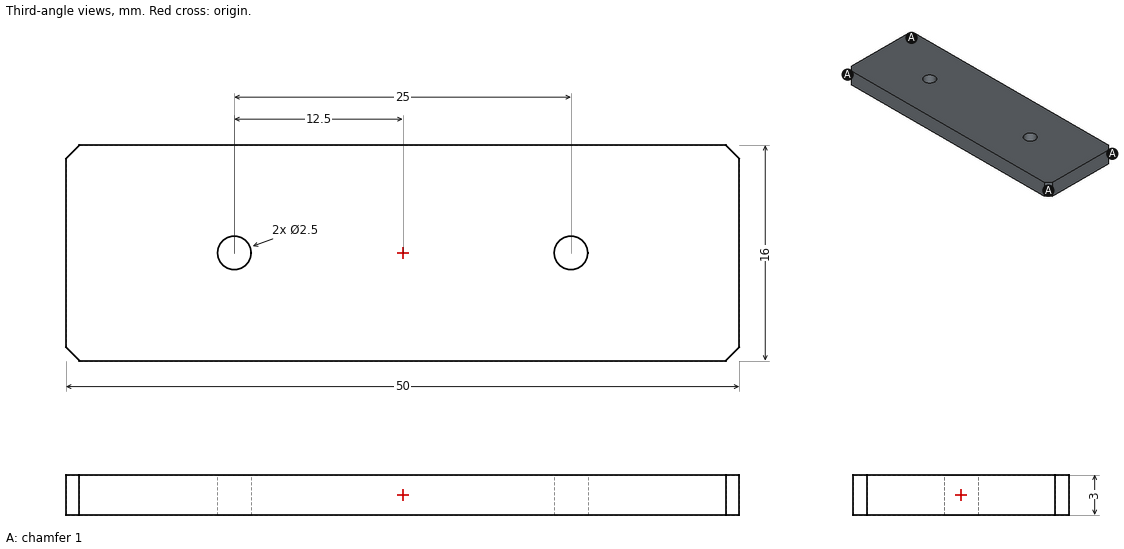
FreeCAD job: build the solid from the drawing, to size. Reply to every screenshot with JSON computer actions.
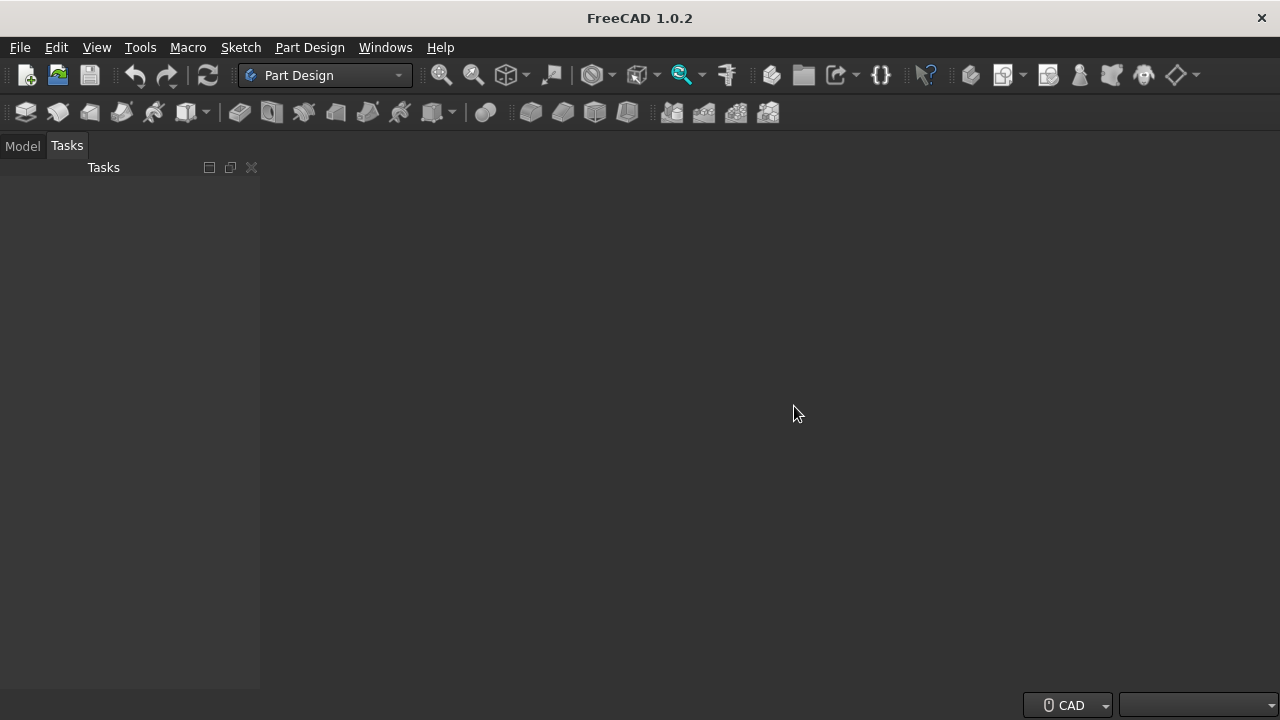
{"action": "left_click", "coordinate": [26, 76]}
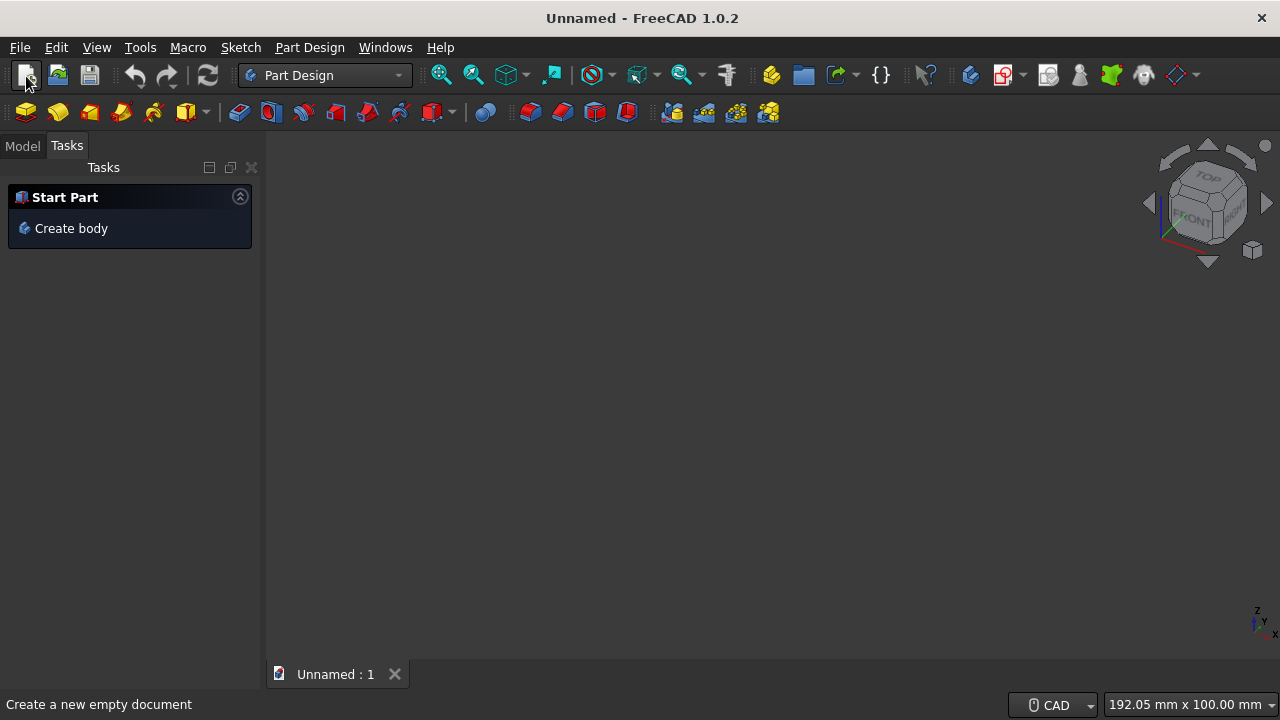
{"action": "left_click", "coordinate": [1004, 76]}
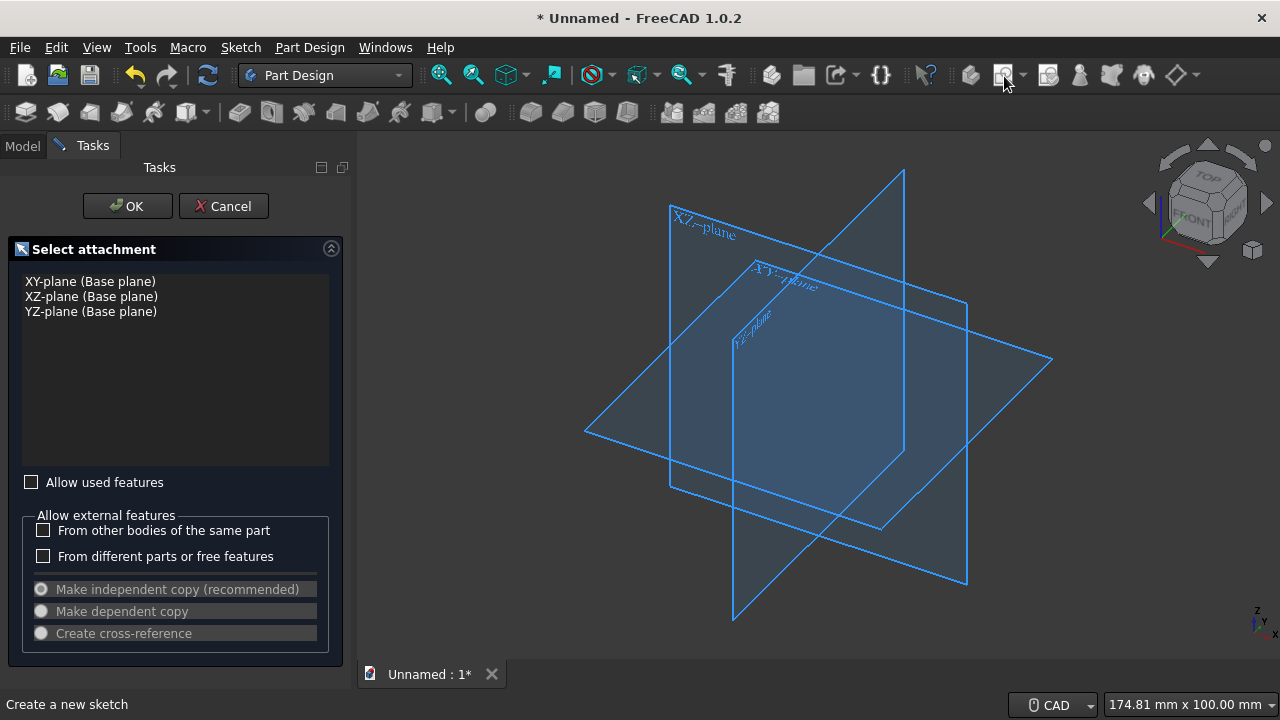
{"action": "left_click", "coordinate": [82, 282]}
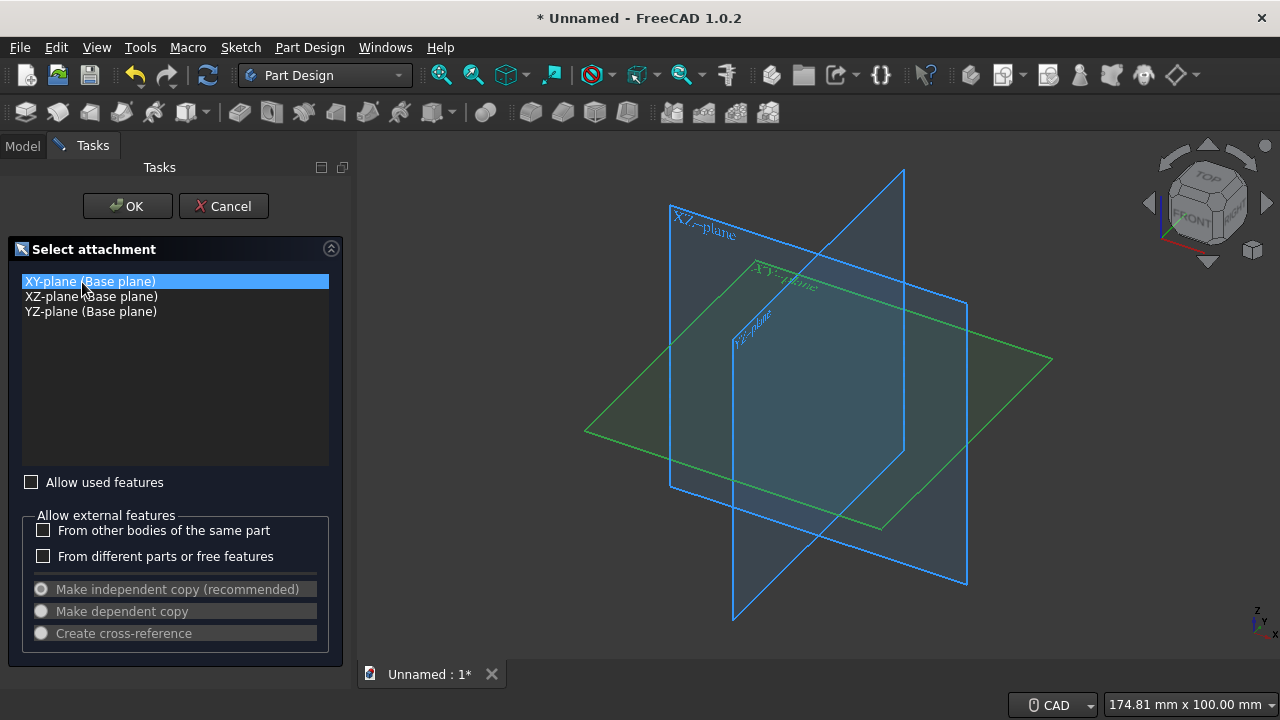
{"action": "left_click", "coordinate": [128, 206]}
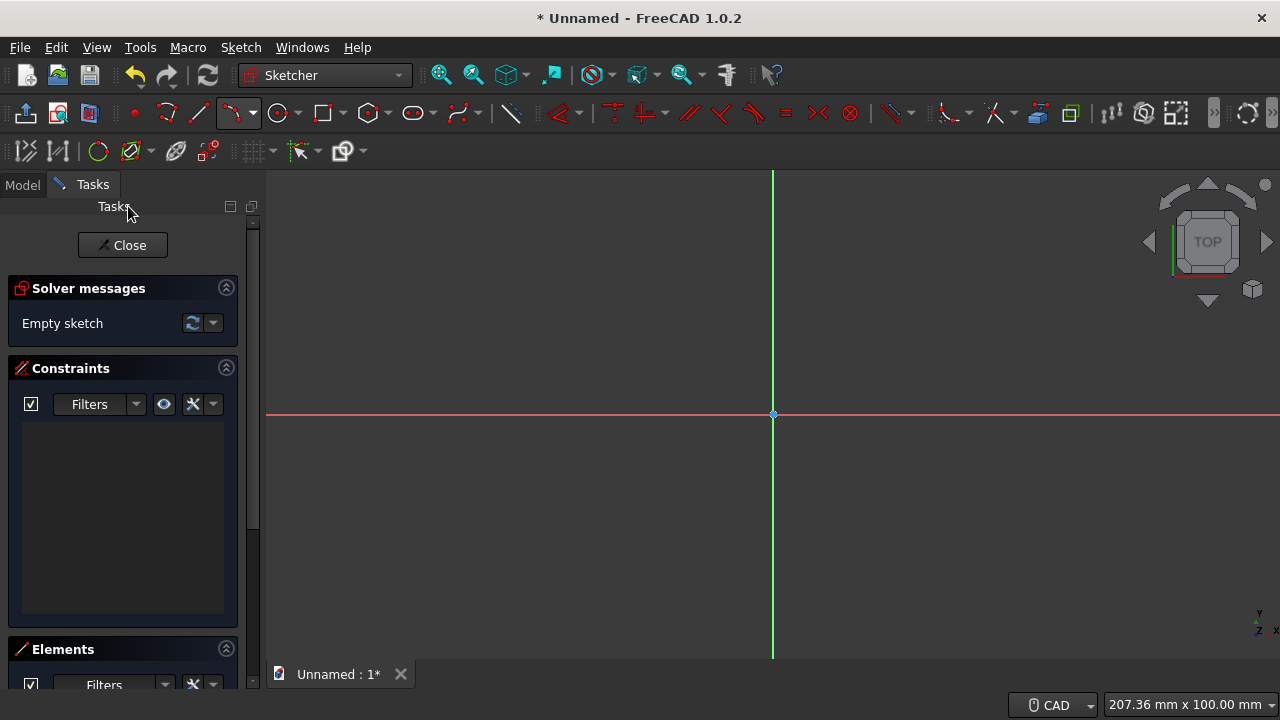
{"action": "scroll", "coordinate": [829, 414], "scroll_direction": "up", "scroll_amount": 4}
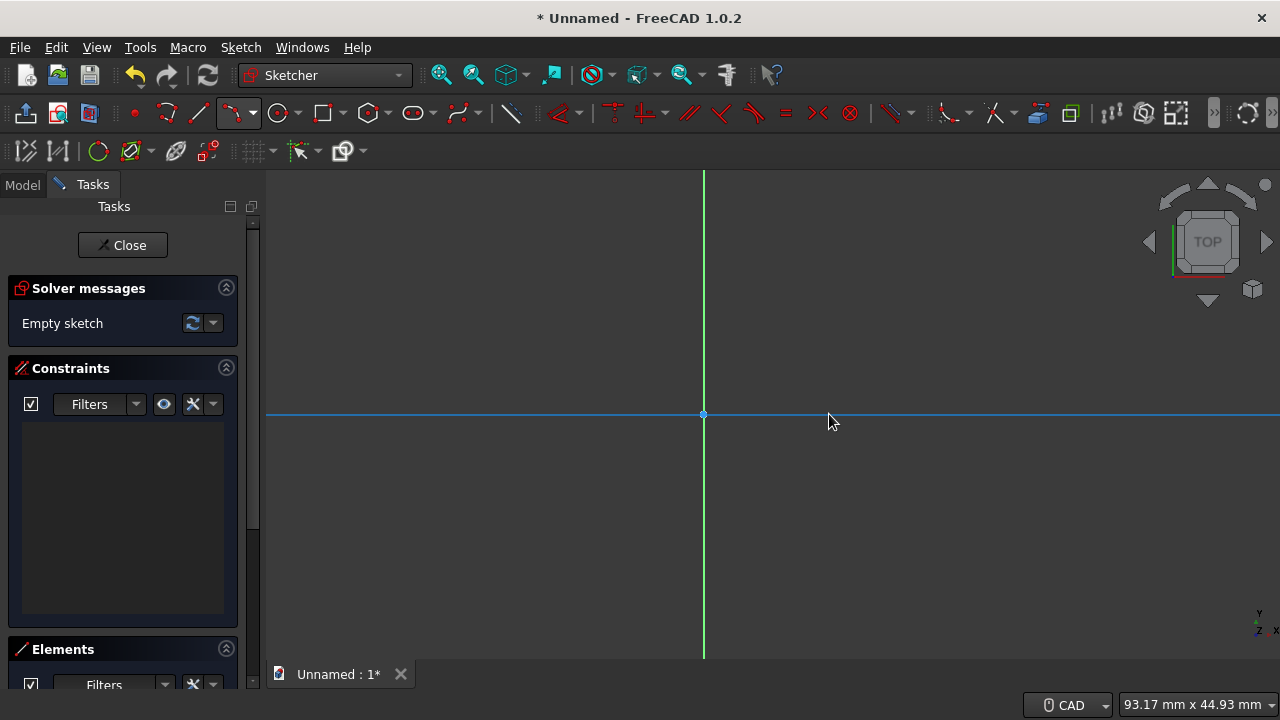
{"action": "key", "text": "g v"}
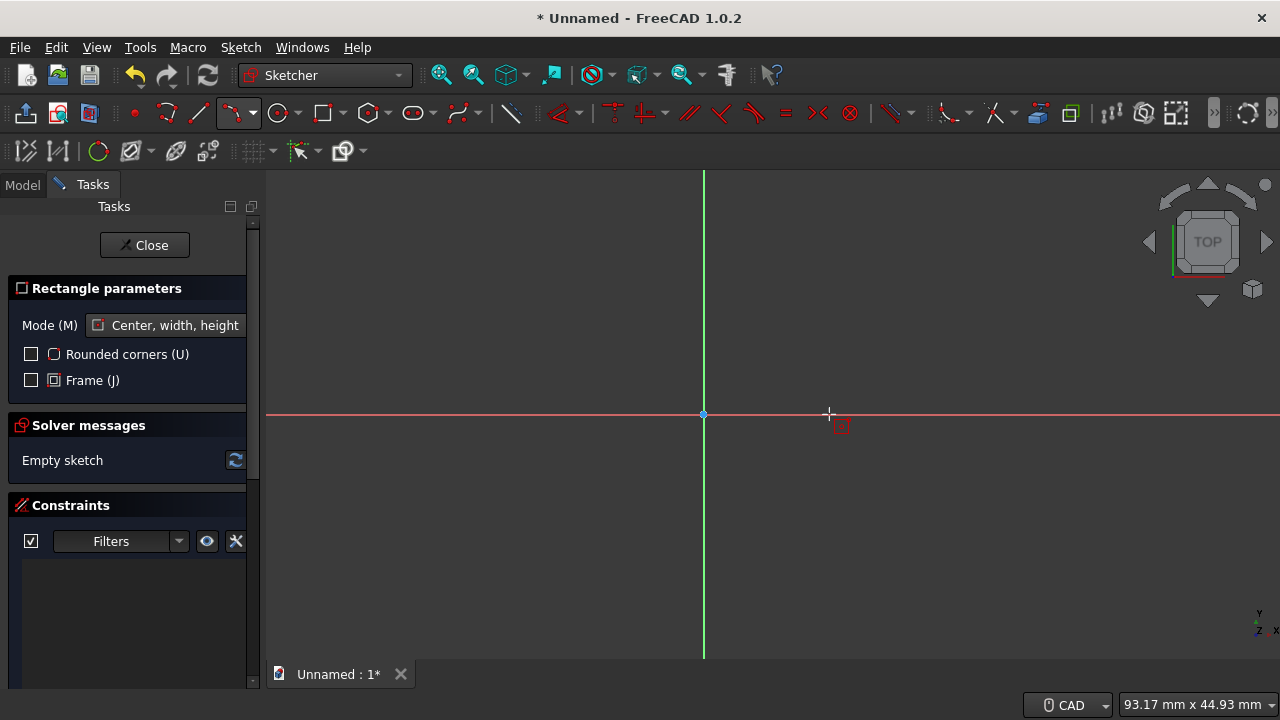
{"action": "left_click", "coordinate": [704, 414]}
{"action": "left_click", "coordinate": [976, 327]}
{"action": "key", "text": "Escape"}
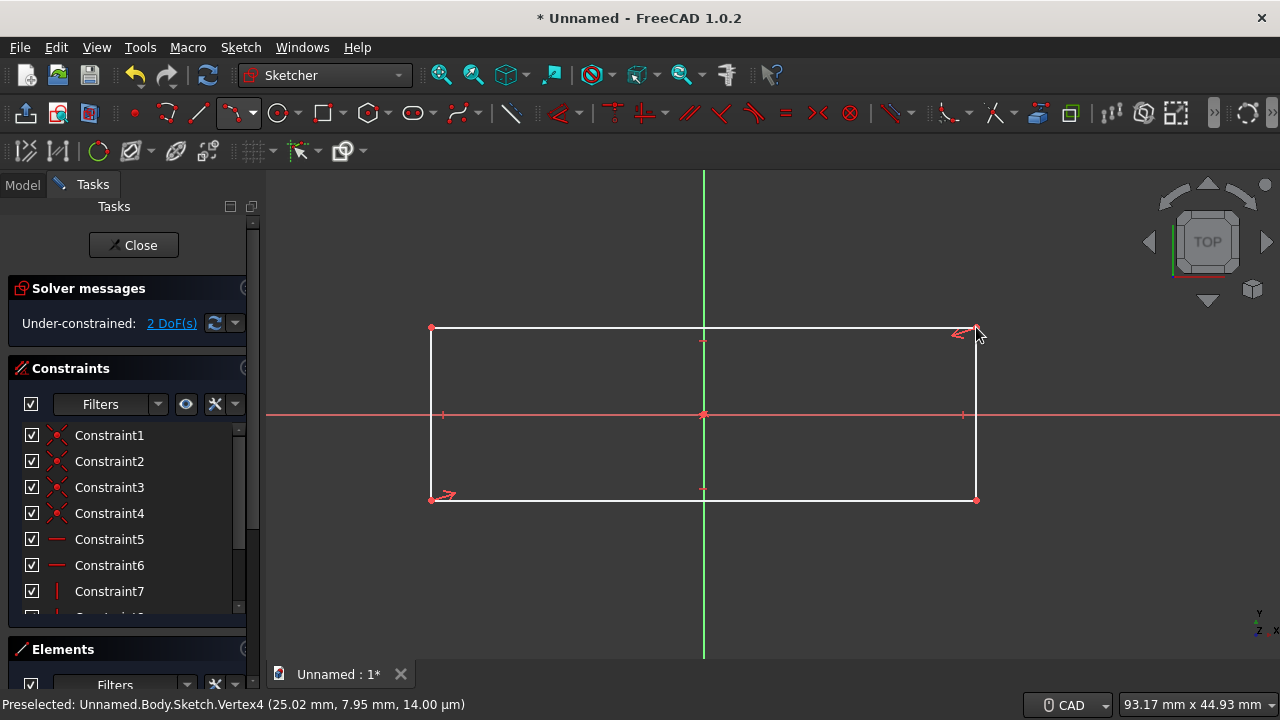
{"action": "left_click", "coordinate": [558, 114]}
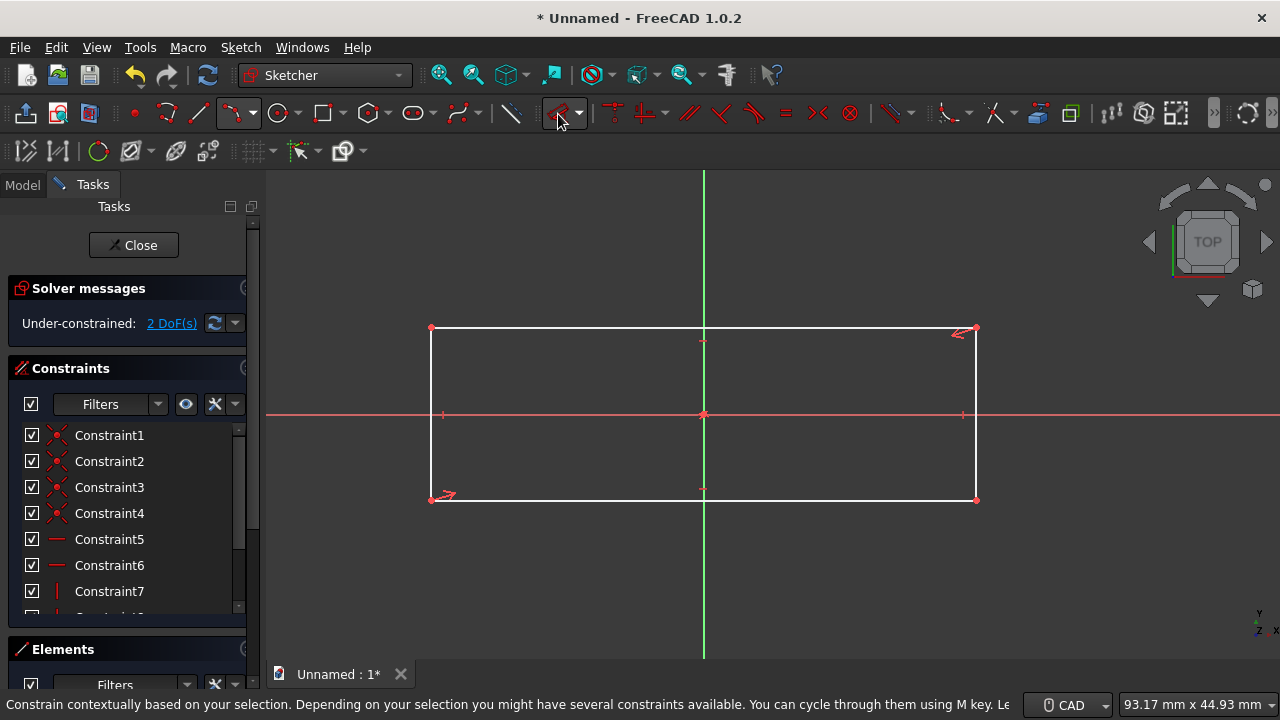
{"action": "left_click", "coordinate": [595, 501]}
{"action": "left_click", "coordinate": [578, 535]}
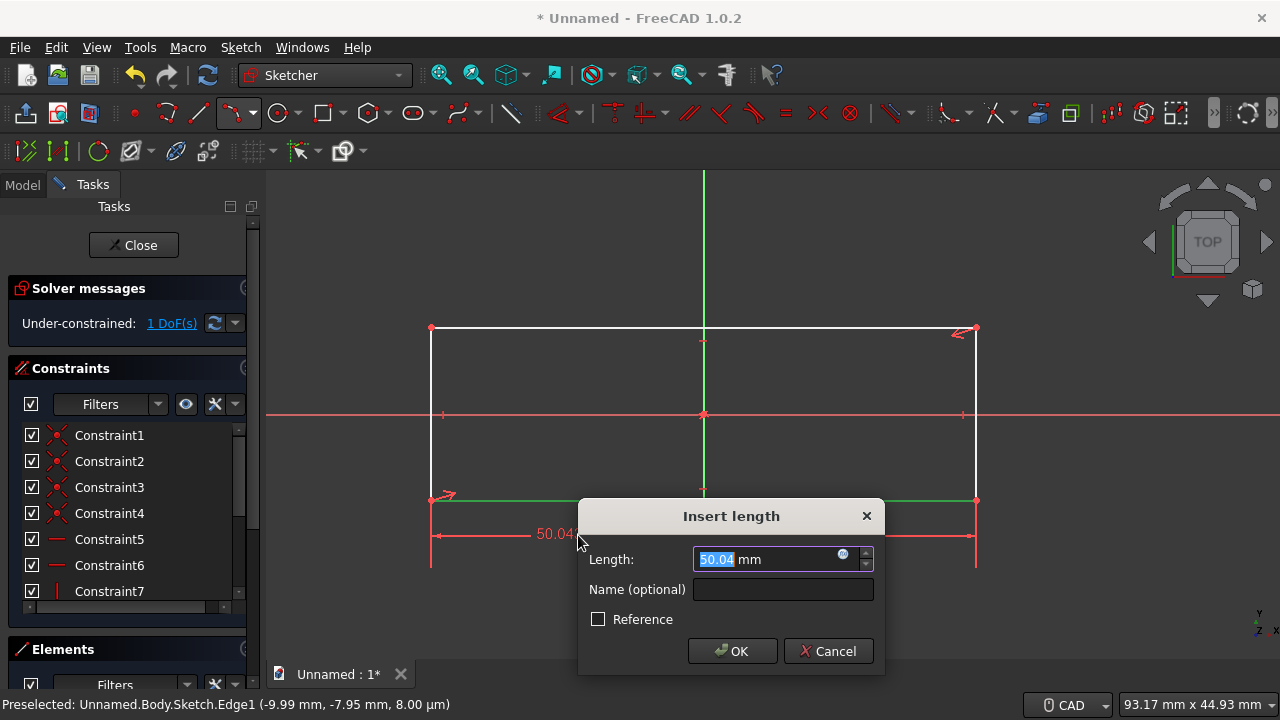
{"action": "type", "text": "50"}
{"action": "key", "text": "Return"}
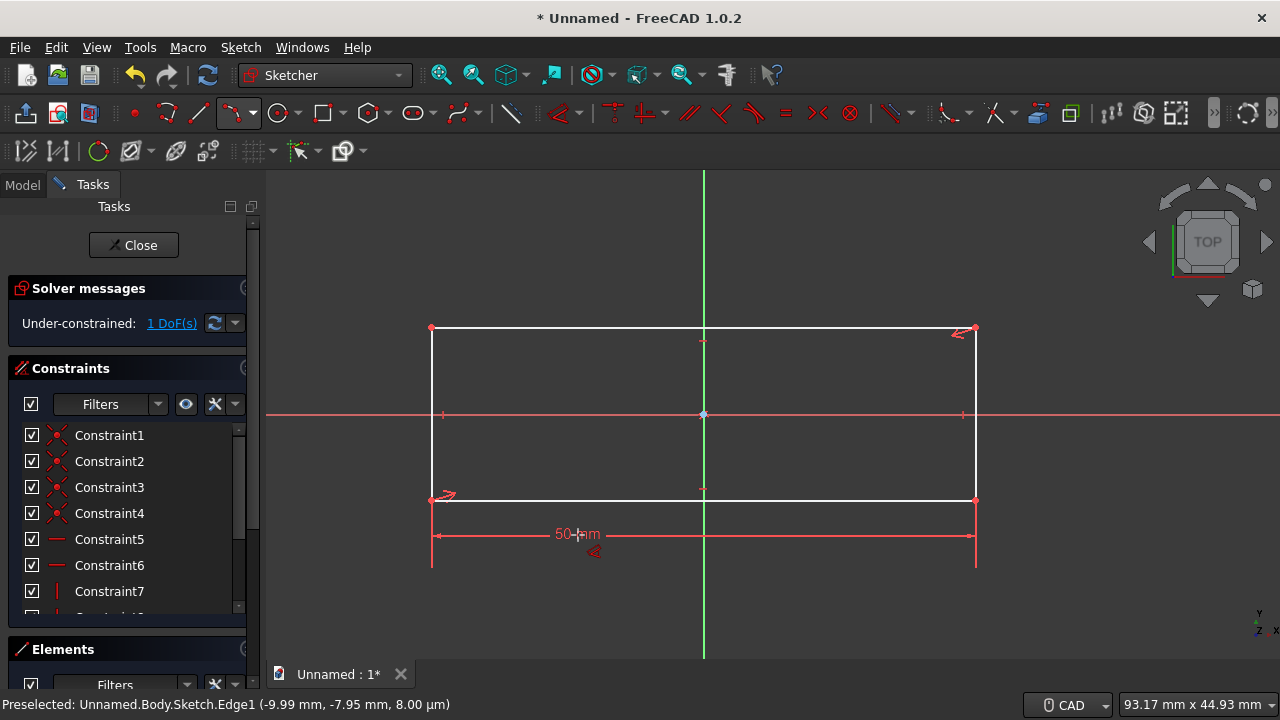
{"action": "left_click", "coordinate": [976, 449]}
{"action": "left_click", "coordinate": [1010, 375]}